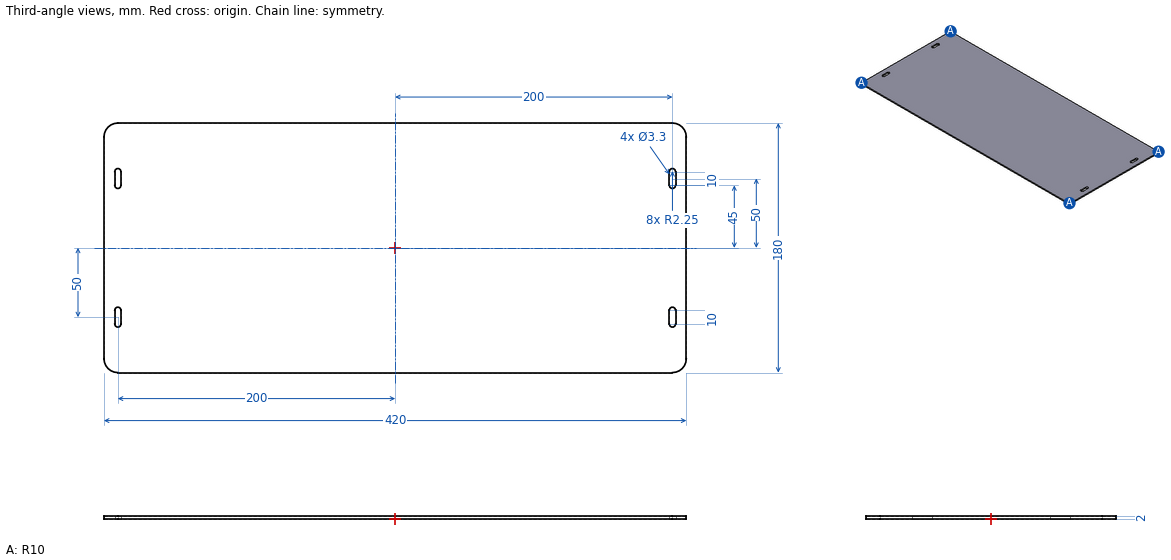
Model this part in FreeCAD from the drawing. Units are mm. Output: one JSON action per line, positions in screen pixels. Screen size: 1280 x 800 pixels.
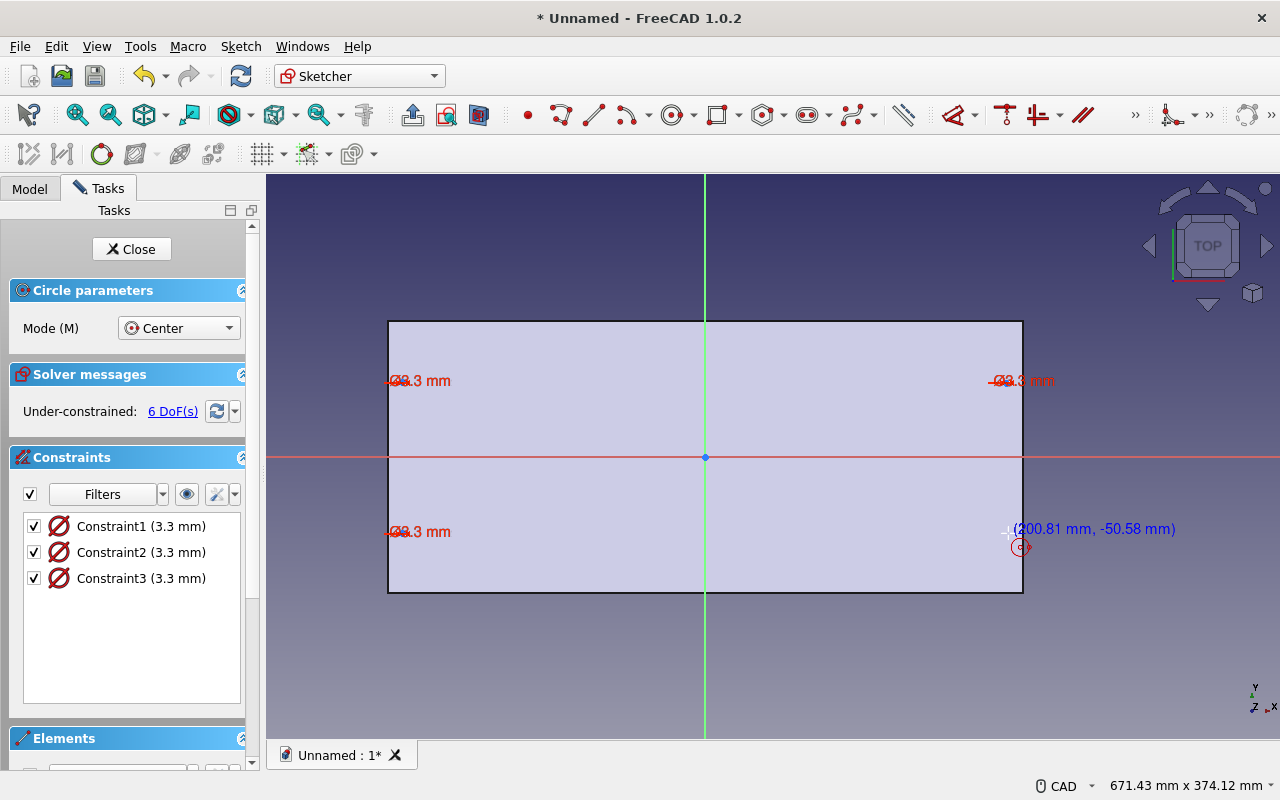
{"action": "left_click", "coordinate": [1007, 533]}
{"action": "mouse_move", "coordinate": [1009, 531]}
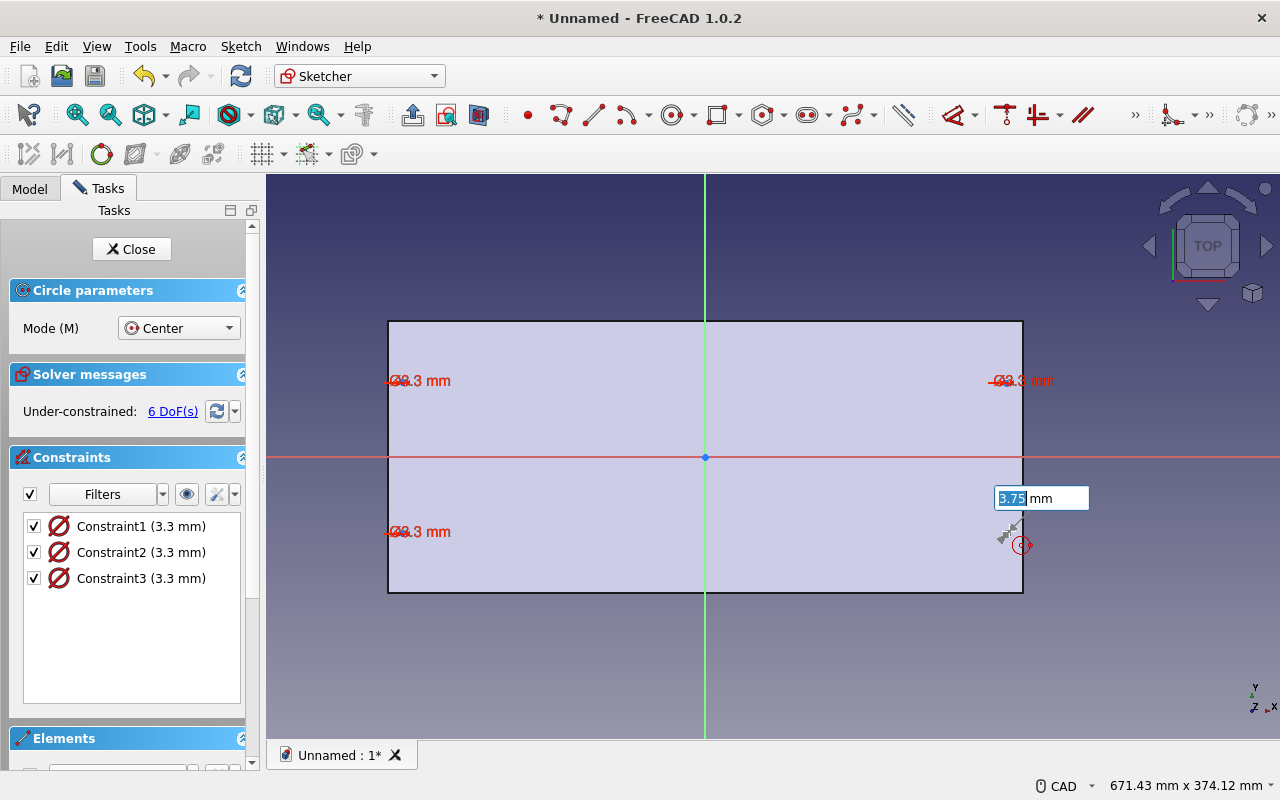
{"action": "type", "text": "3.3"}
{"action": "key", "text": "Return"}
{"action": "key", "text": "Escape"}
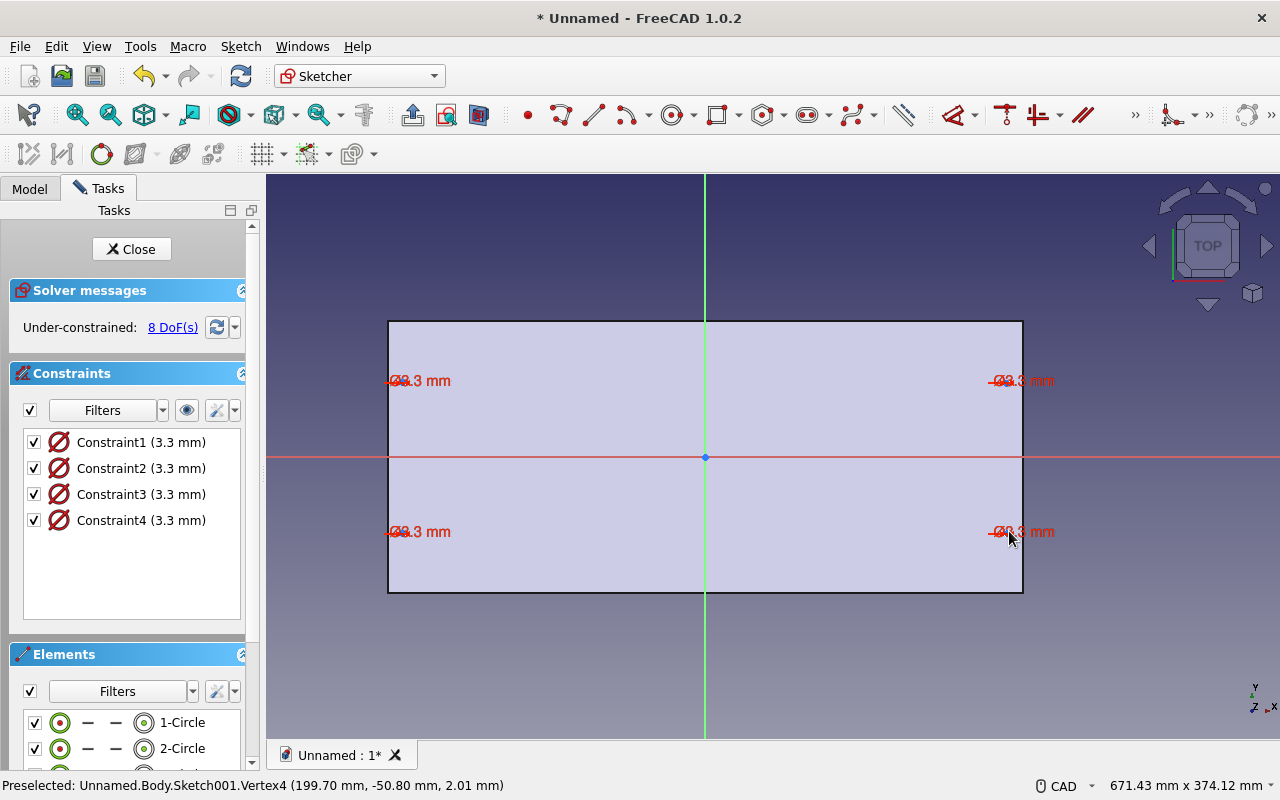
{"action": "left_click", "coordinate": [403, 534]}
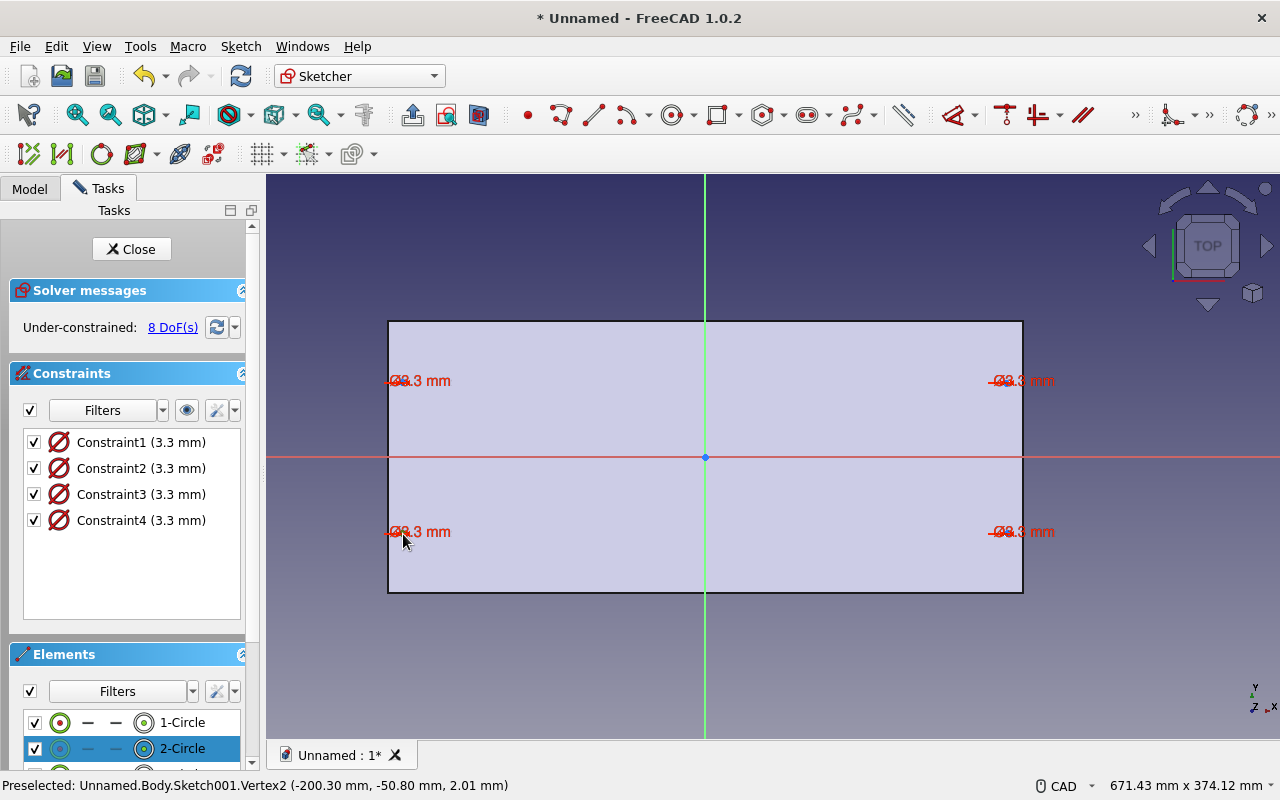
{"action": "left_click", "coordinate": [403, 383]}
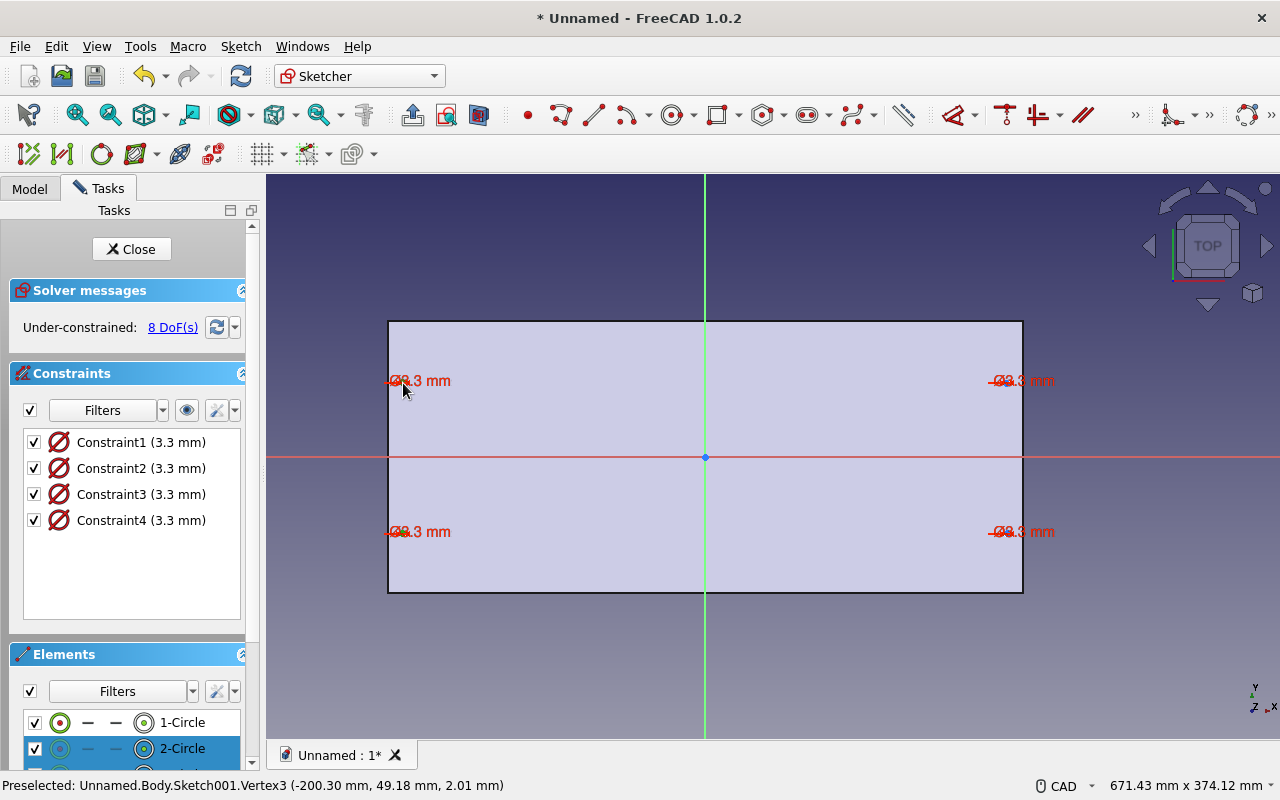
{"action": "left_click", "coordinate": [1060, 116]}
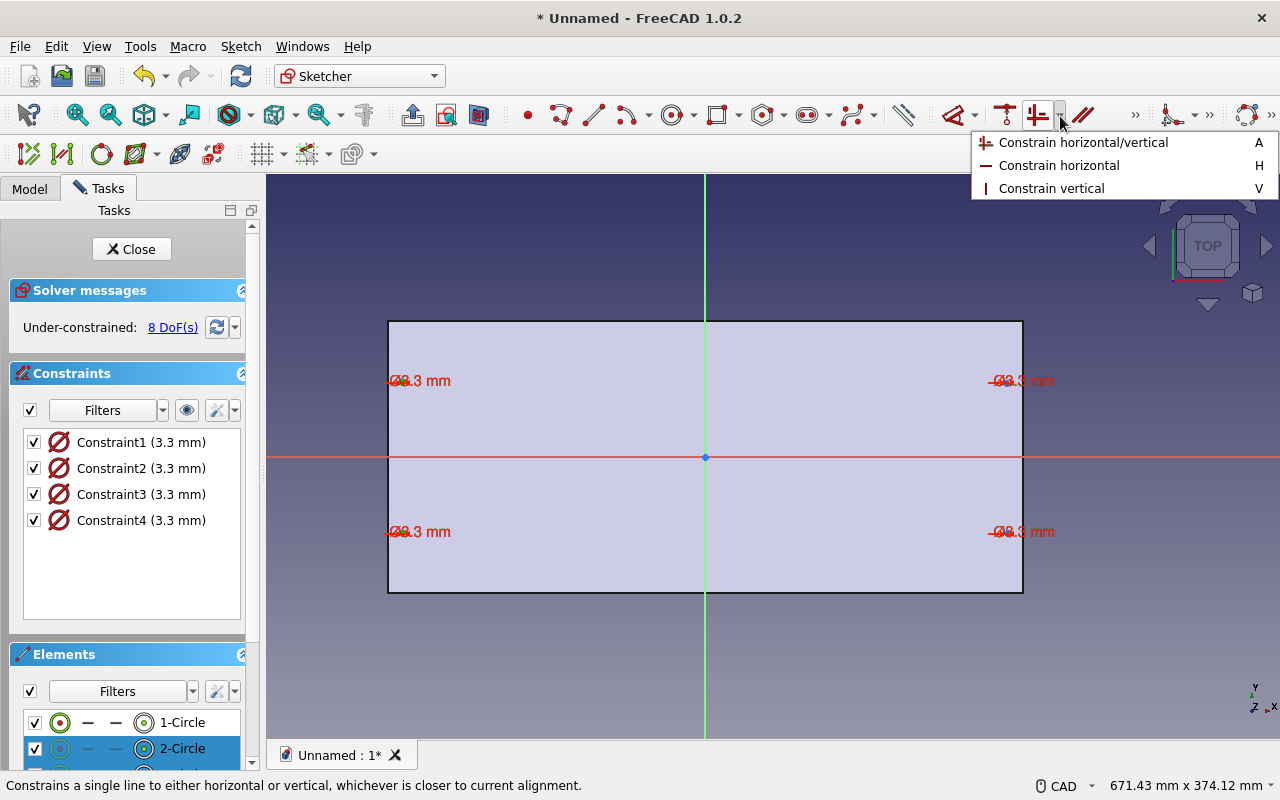
{"action": "left_click", "coordinate": [1125, 188]}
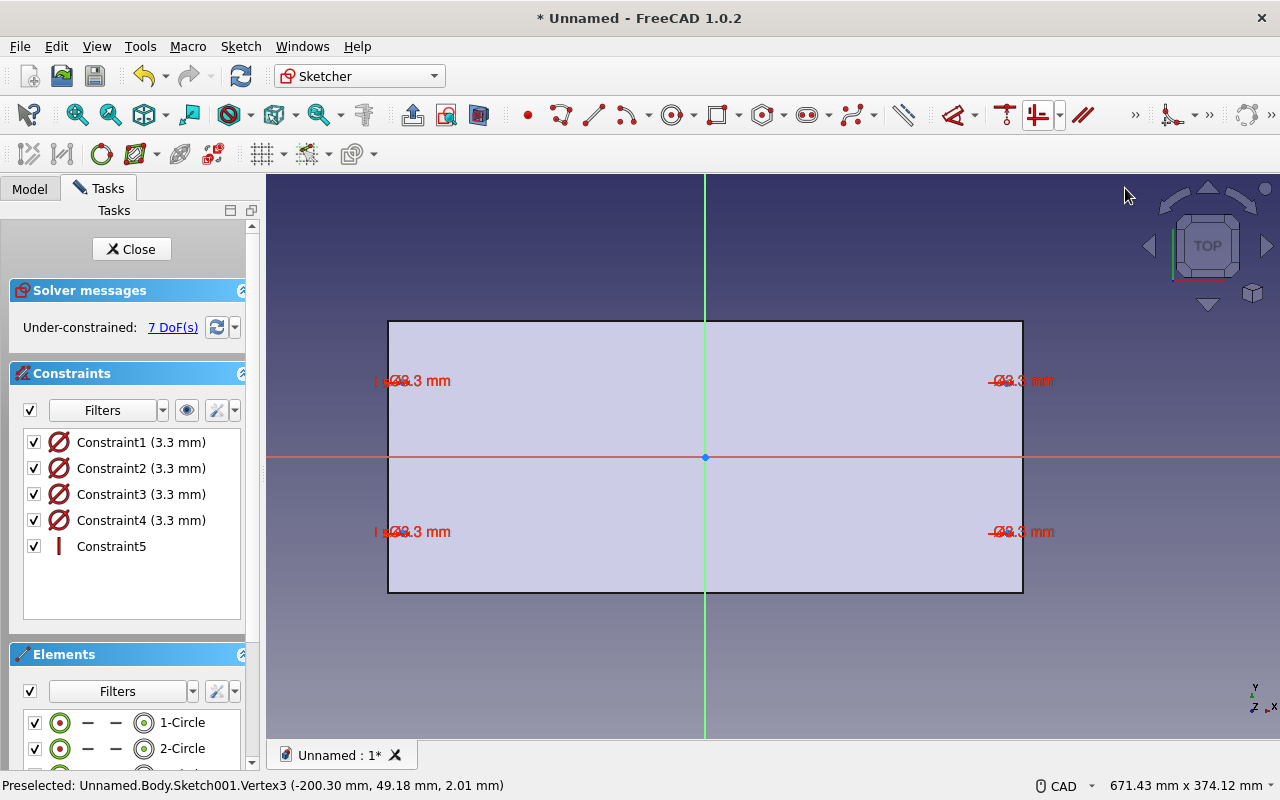
{"action": "left_click", "coordinate": [1007, 383]}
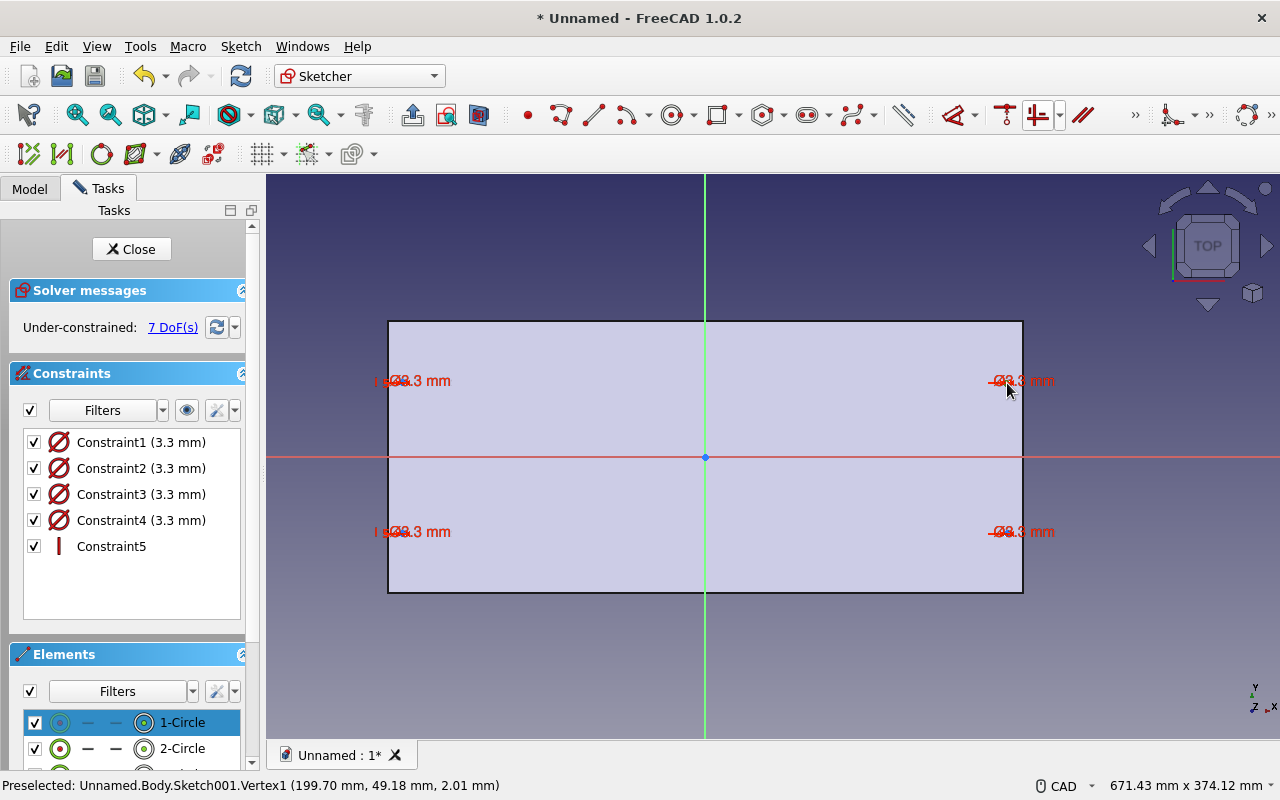
{"action": "left_click", "coordinate": [403, 383]}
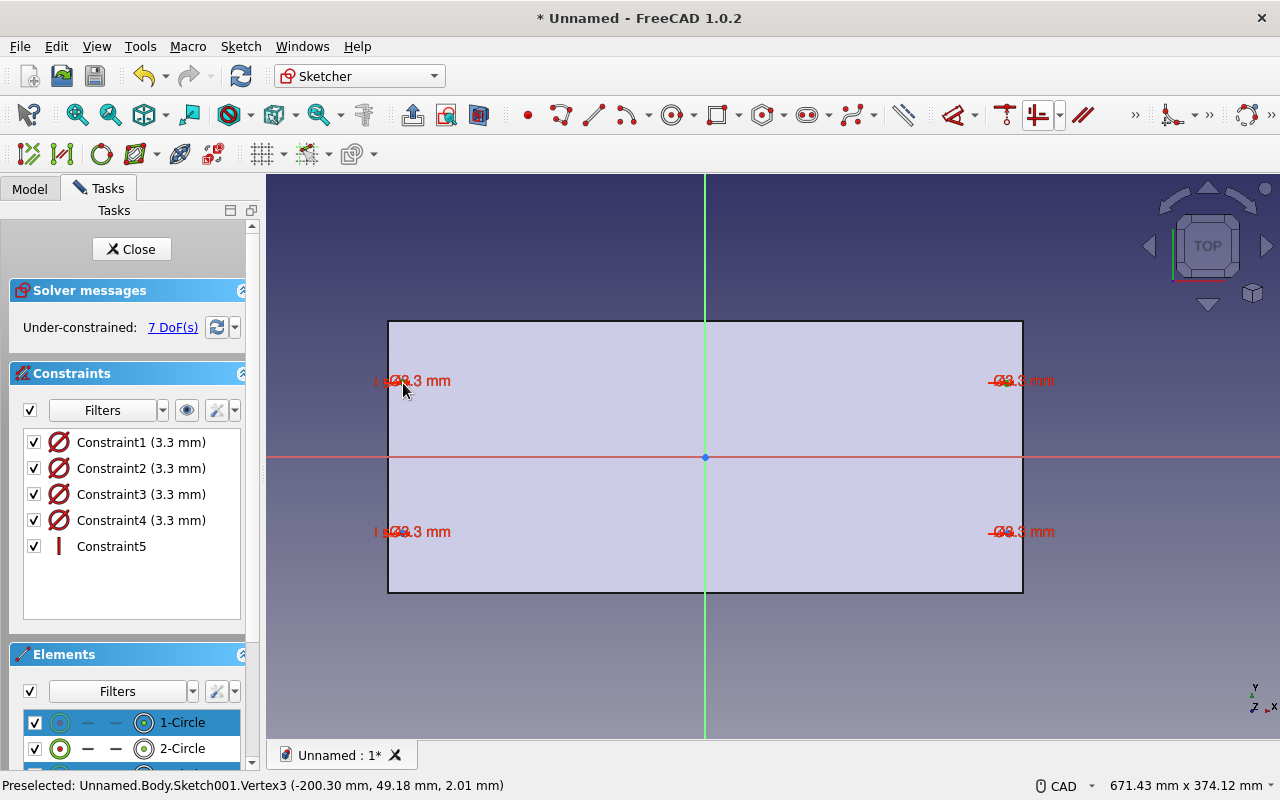
{"action": "left_click", "coordinate": [1060, 116]}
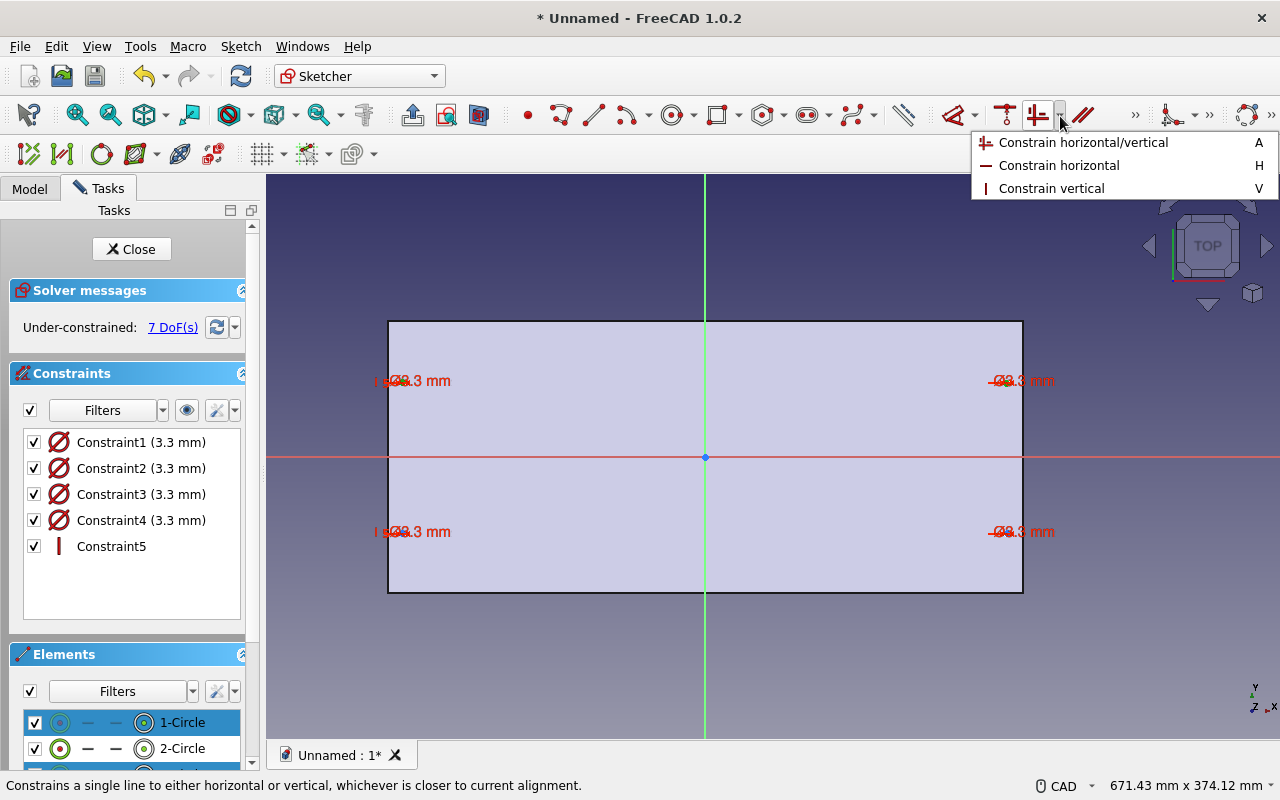
{"action": "left_click", "coordinate": [1125, 166]}